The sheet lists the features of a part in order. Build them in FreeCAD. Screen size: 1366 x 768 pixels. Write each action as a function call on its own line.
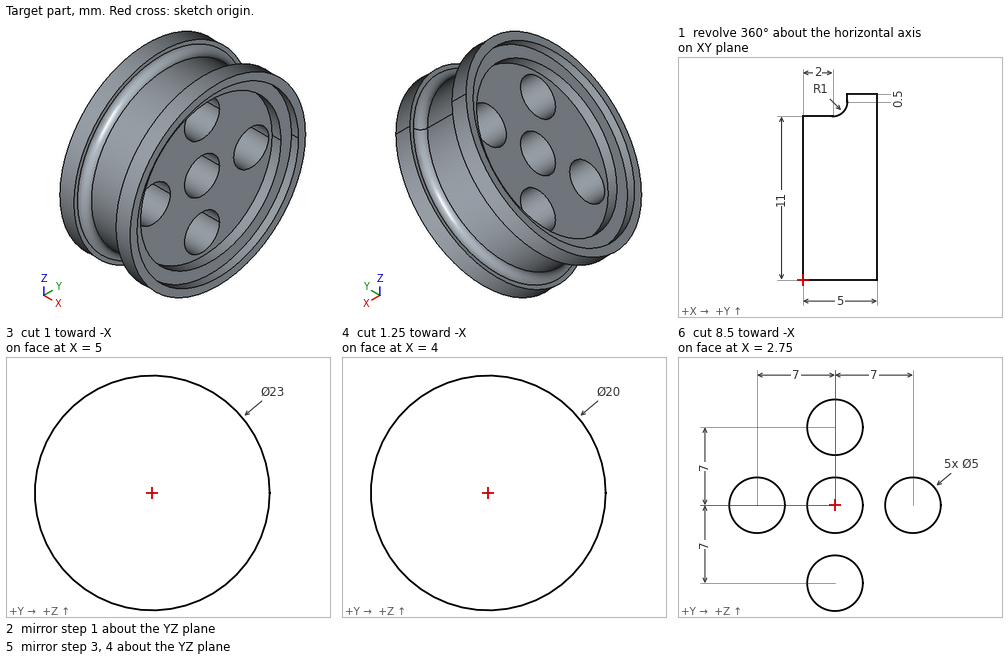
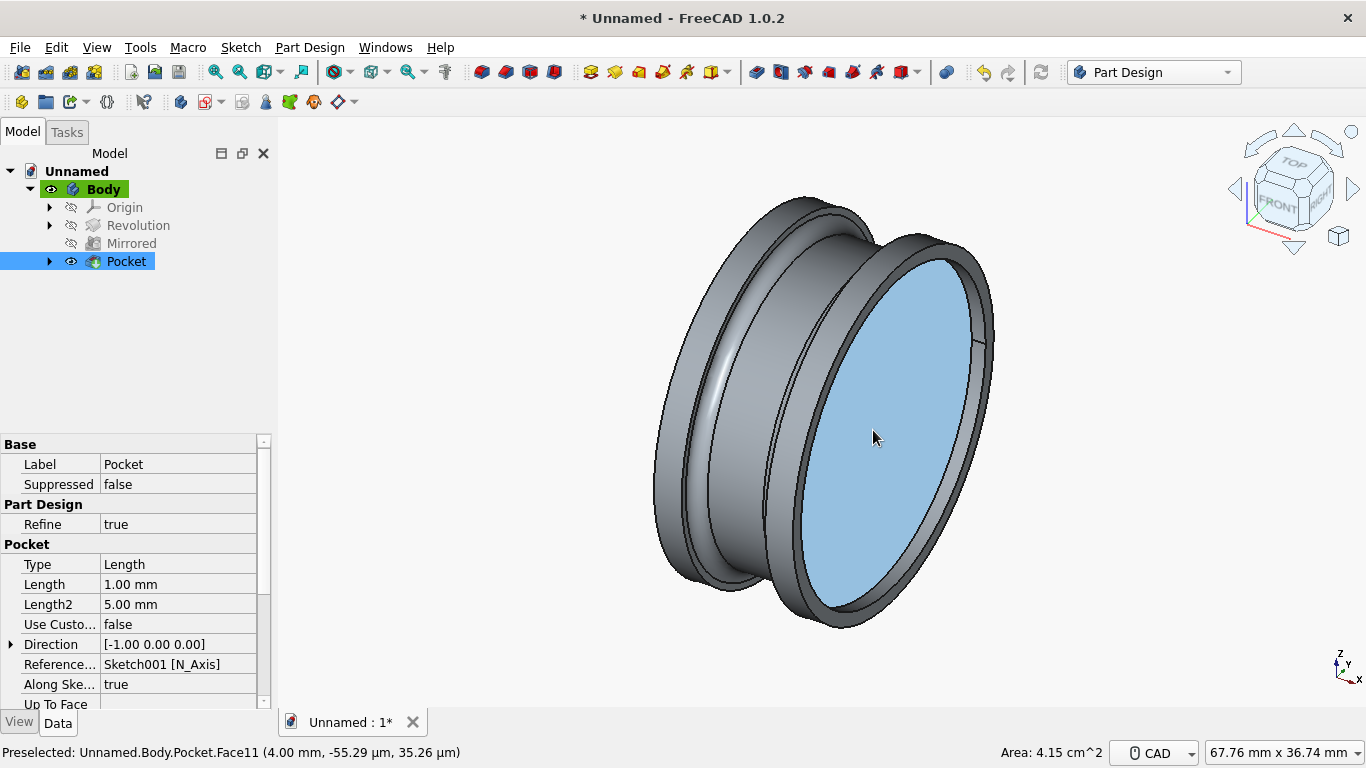
click(206, 102)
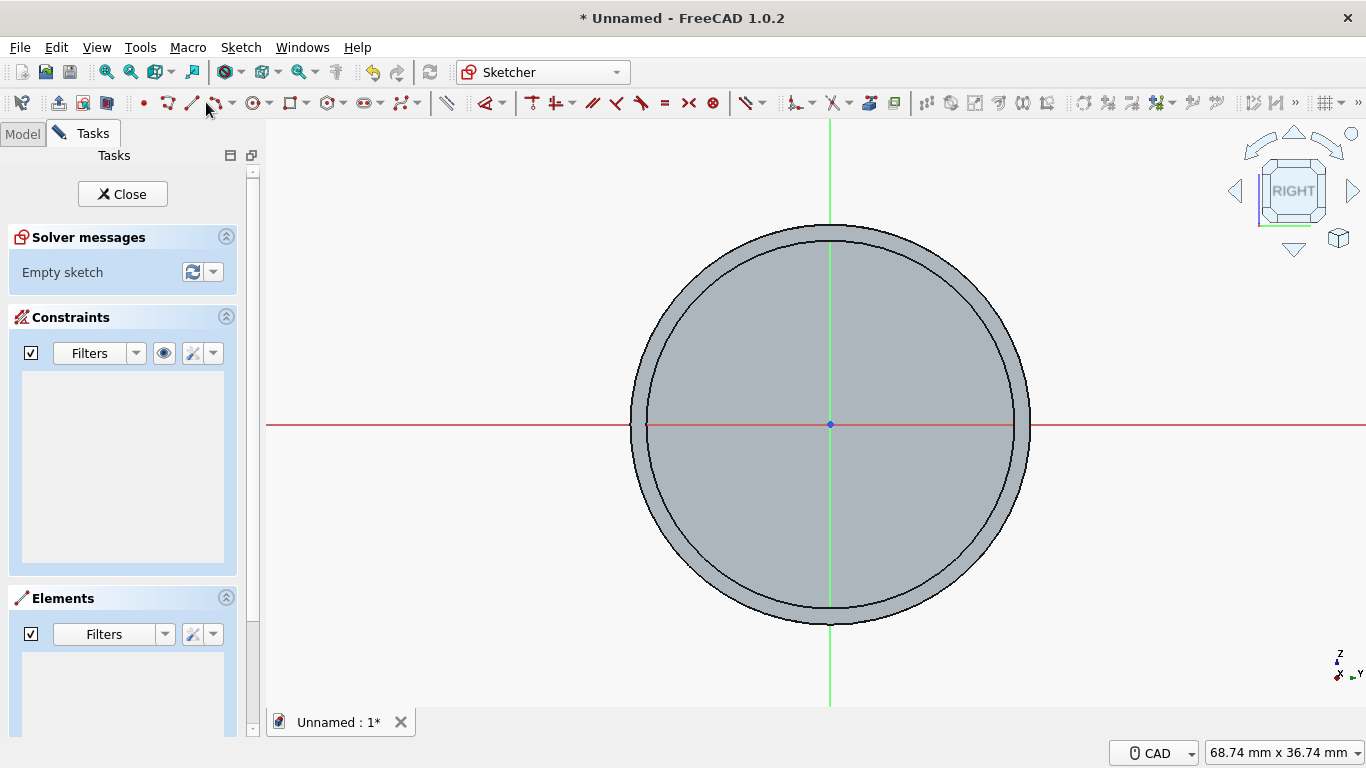
click(108, 104)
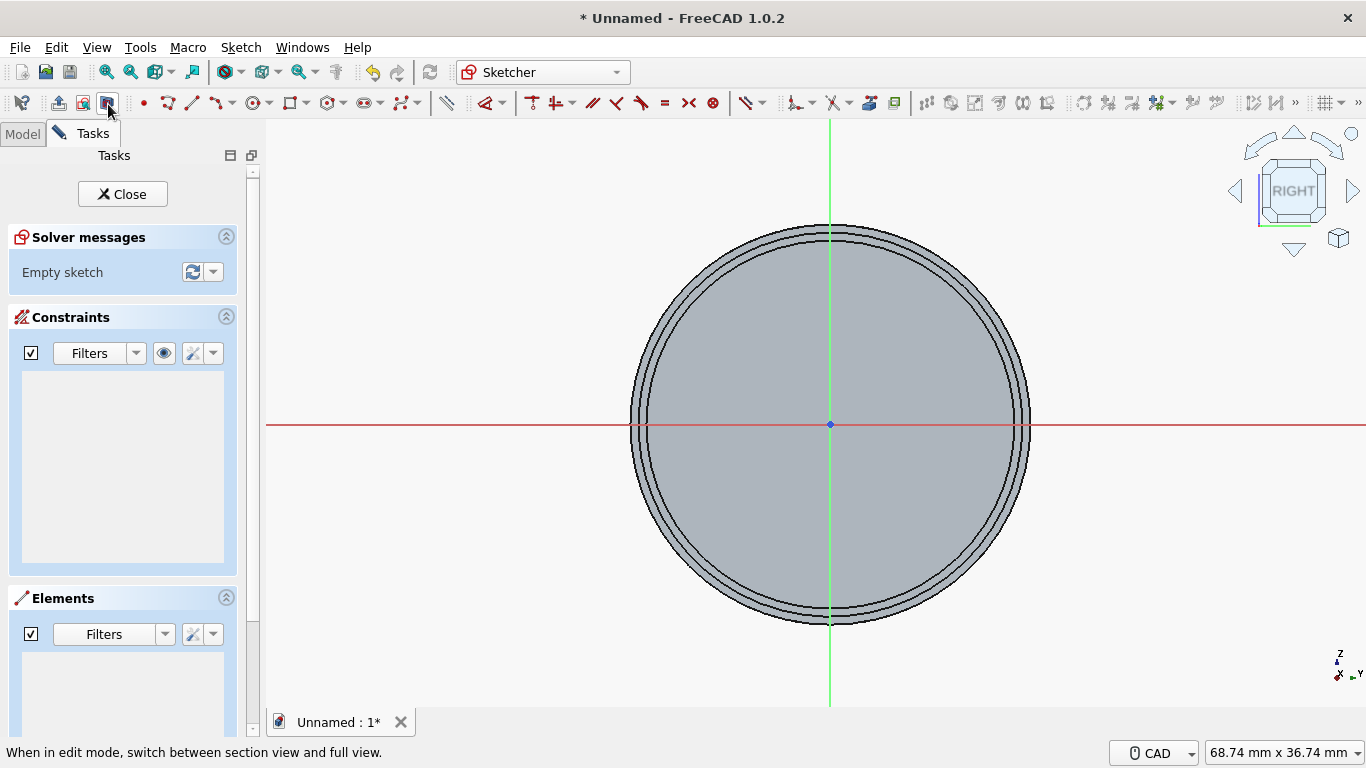
click(254, 104)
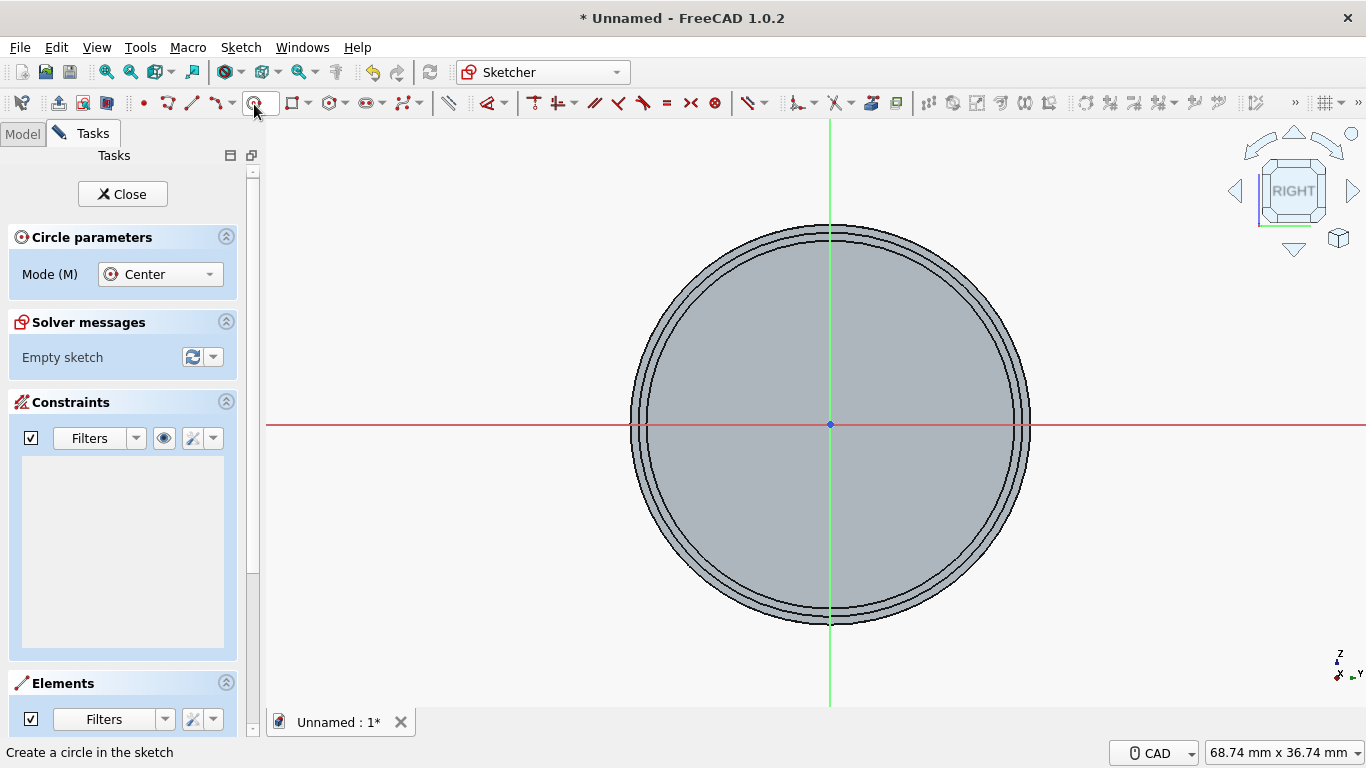
click(830, 425)
click(944, 312)
key(Escape)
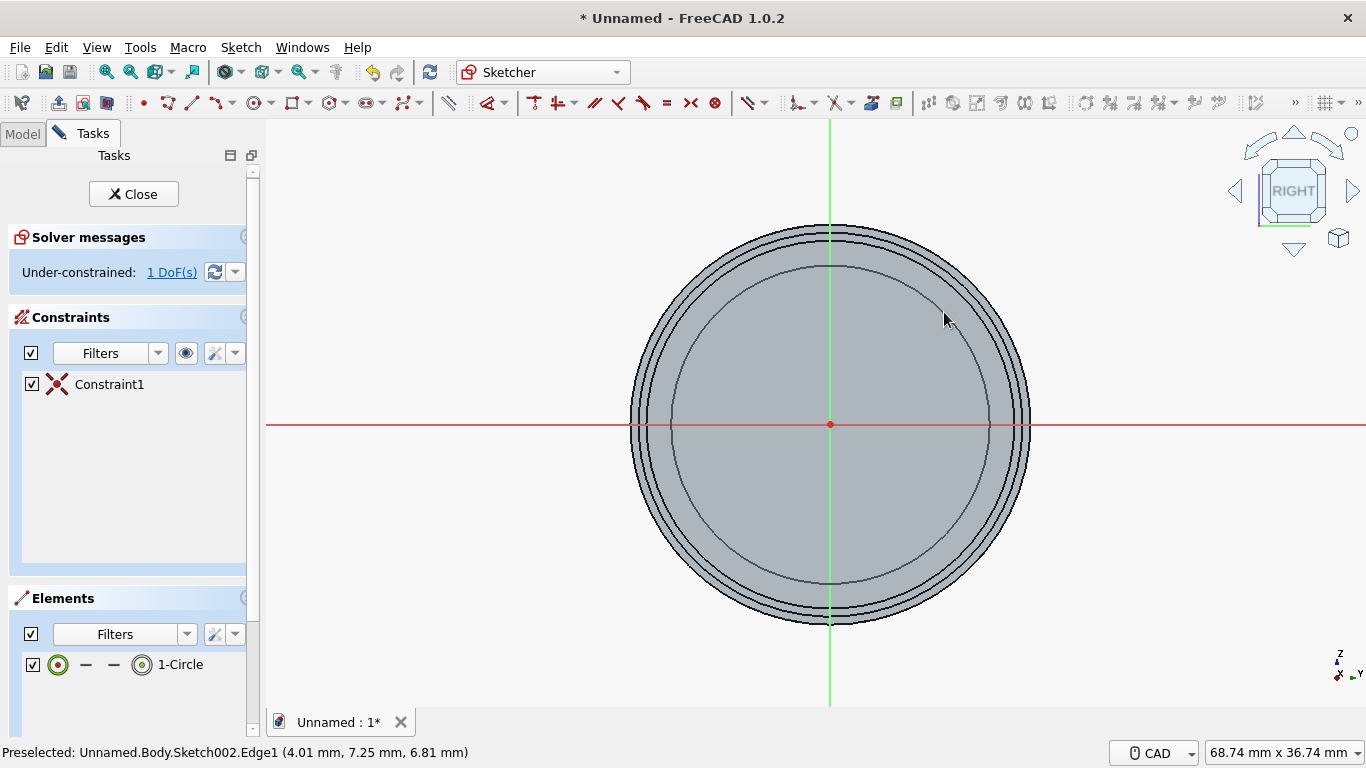
key(d)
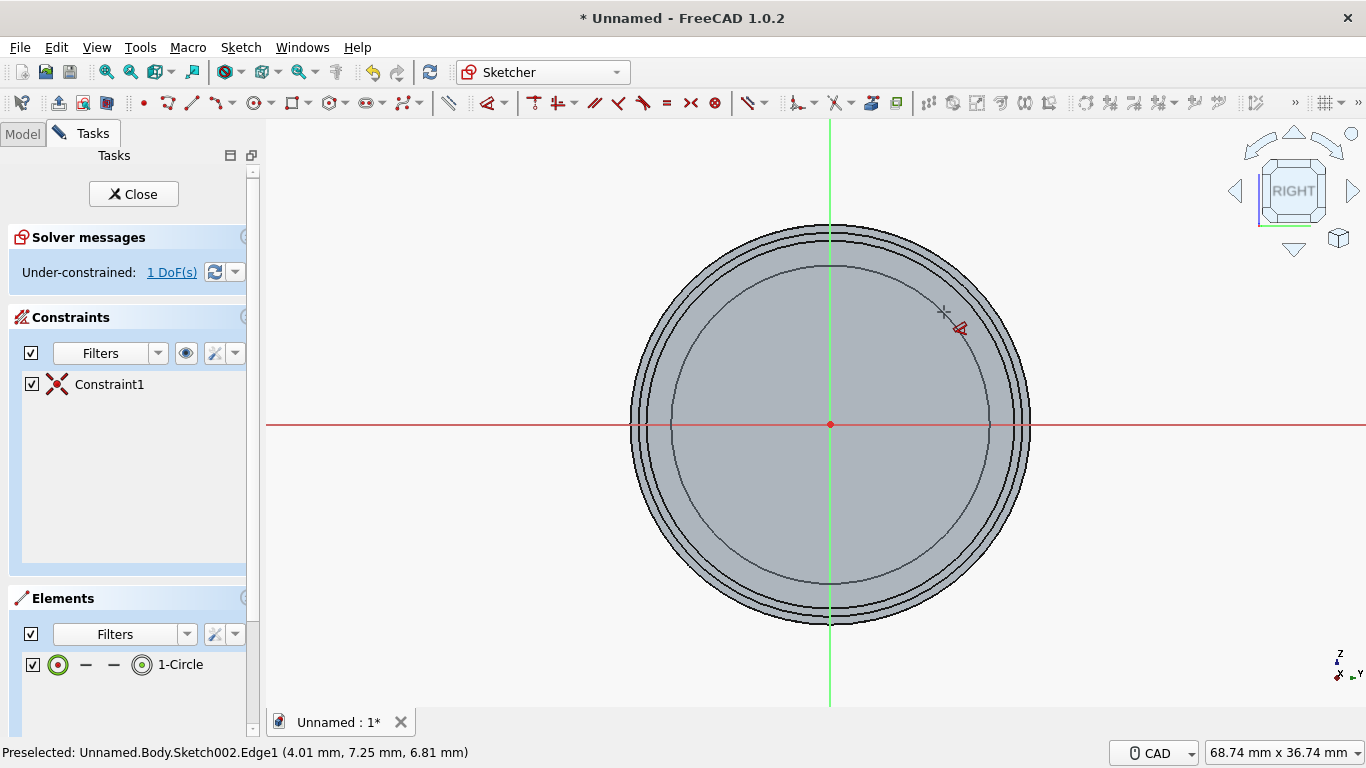
click(943, 312)
click(966, 289)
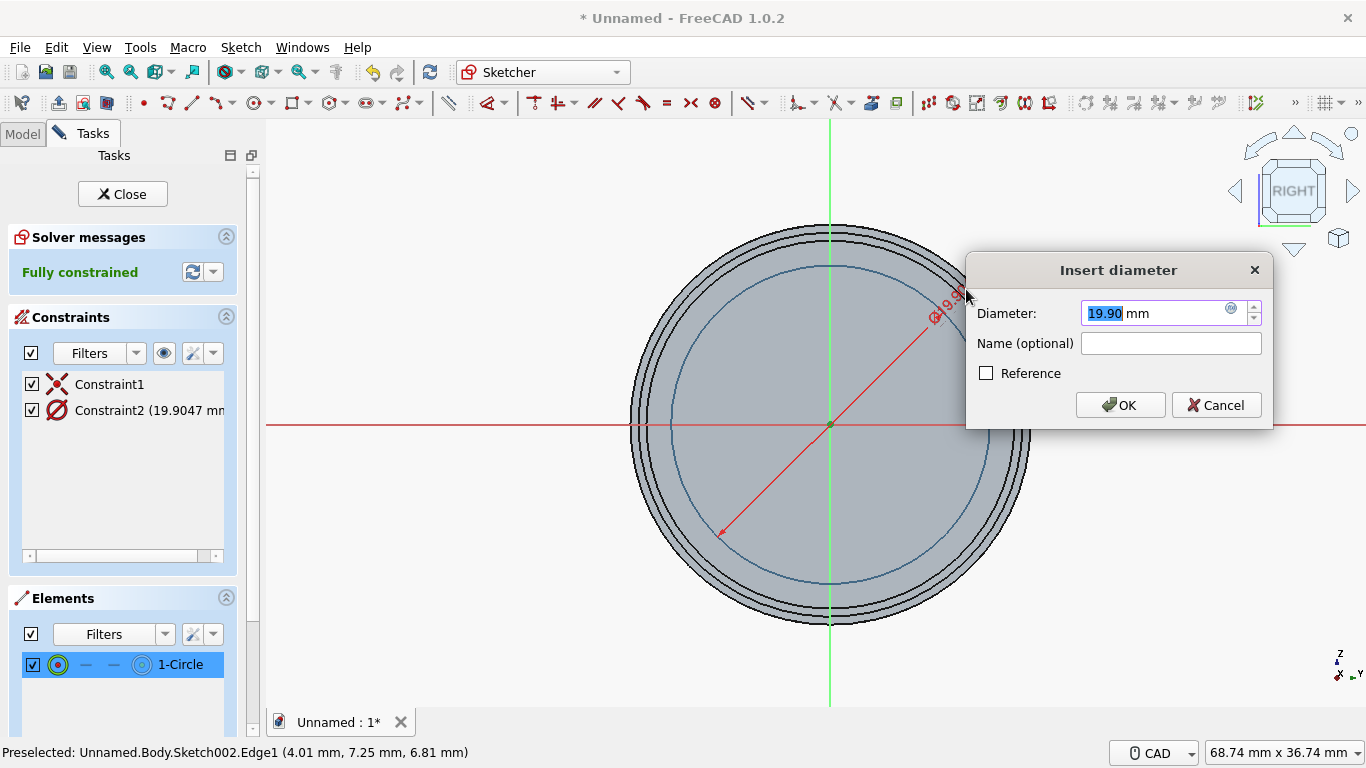
text(20)
key(Return)
key(Escape)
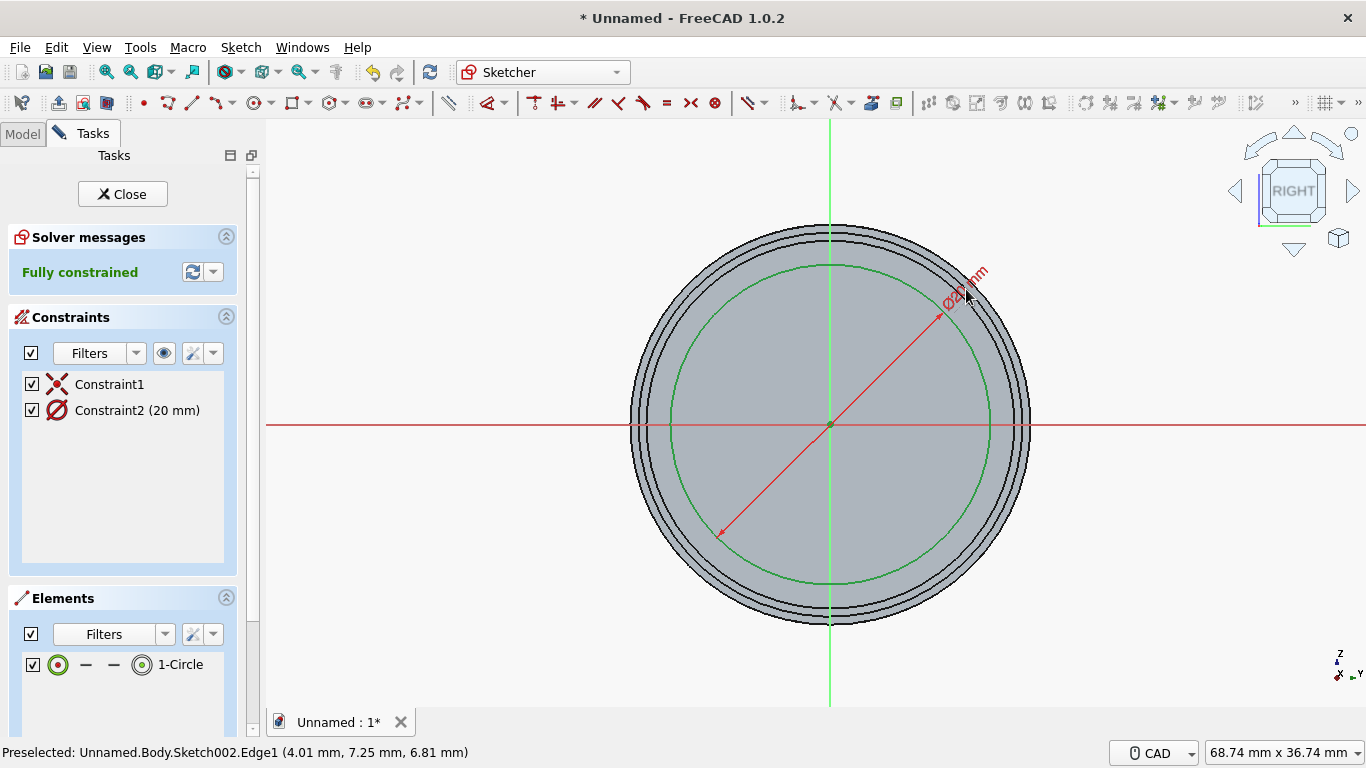
click(123, 194)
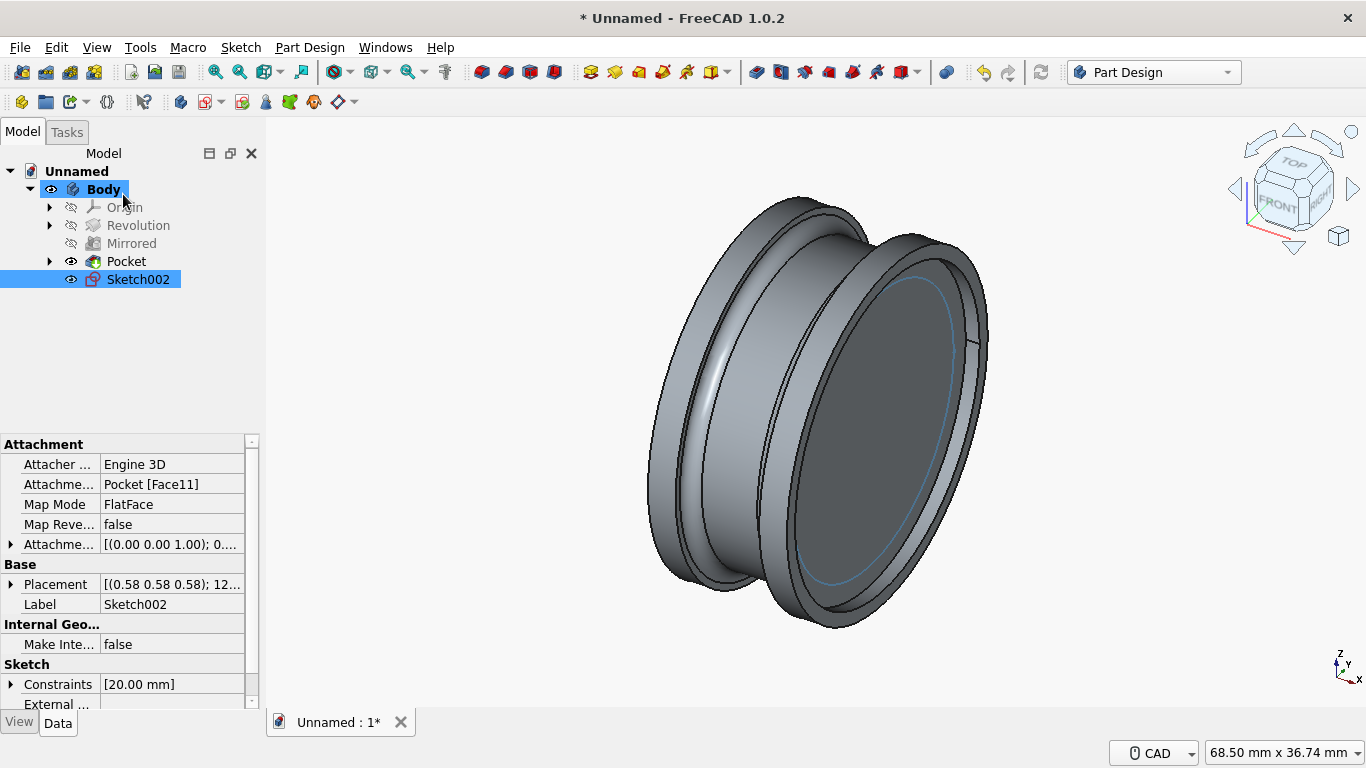
click(758, 72)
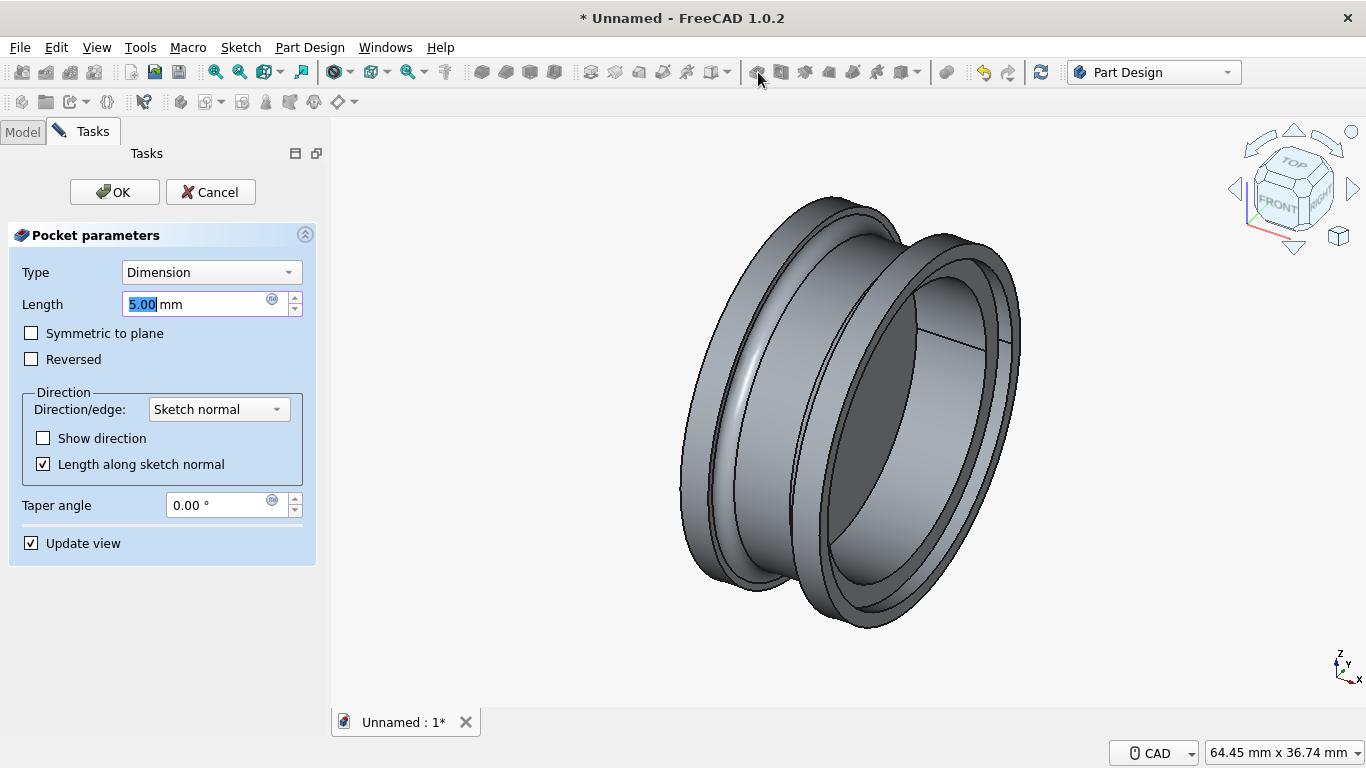
text(1.25)
key(Tab)